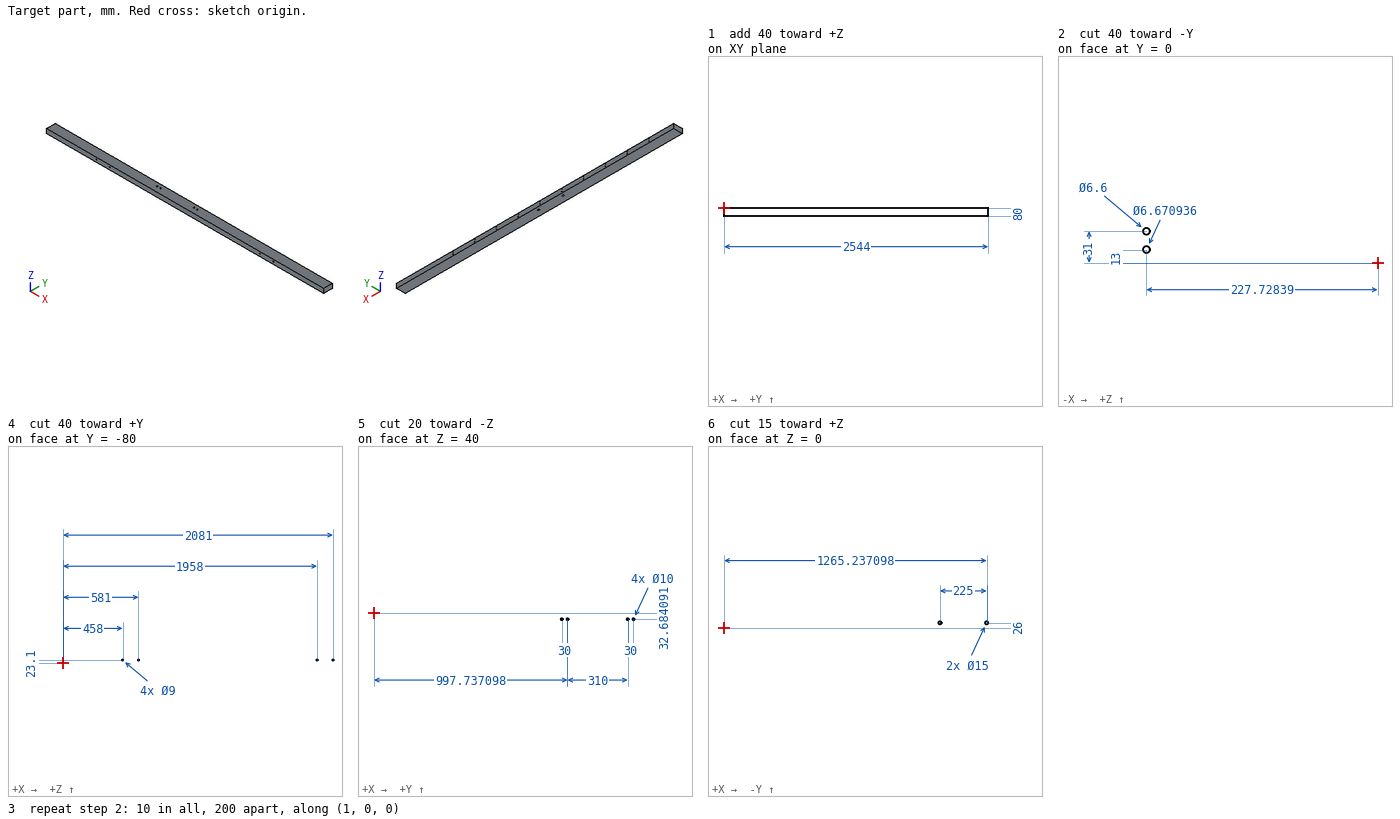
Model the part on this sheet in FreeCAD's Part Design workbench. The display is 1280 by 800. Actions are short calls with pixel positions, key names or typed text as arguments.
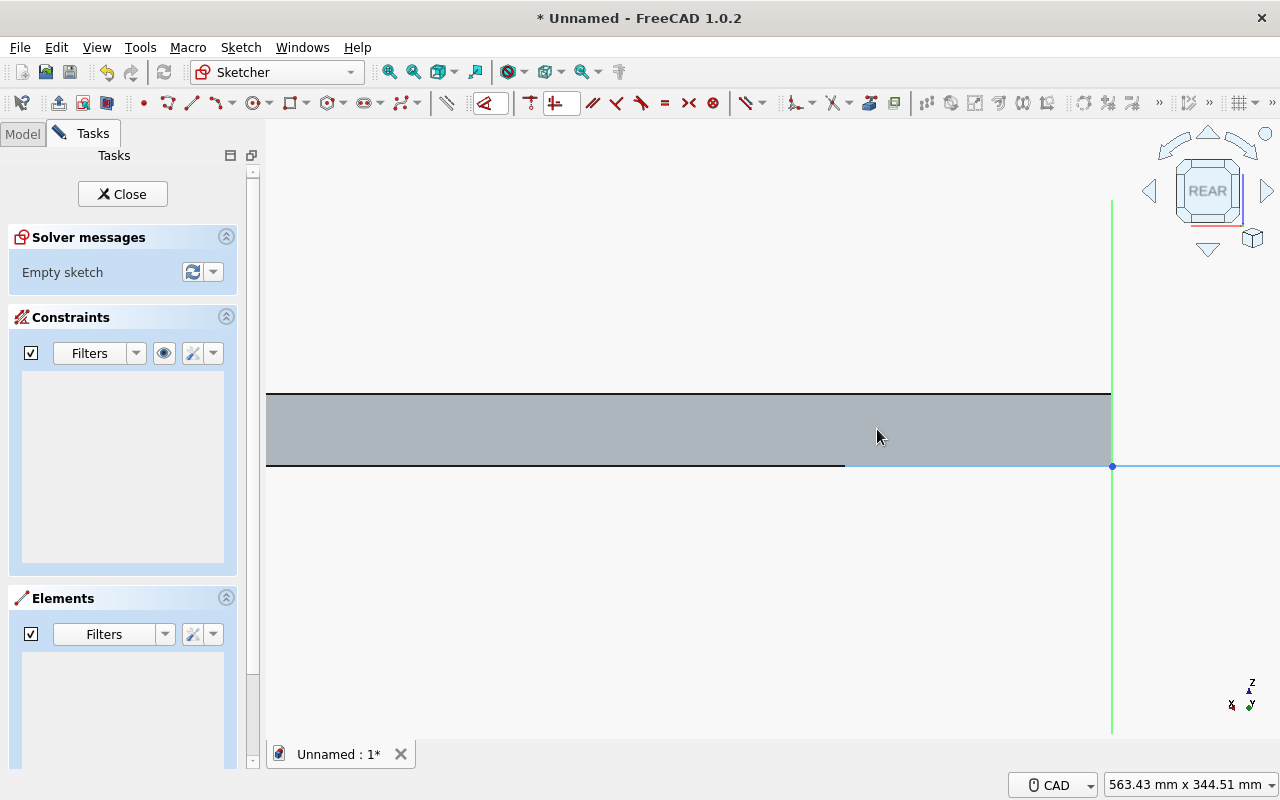
scroll(702, 427, up, 11)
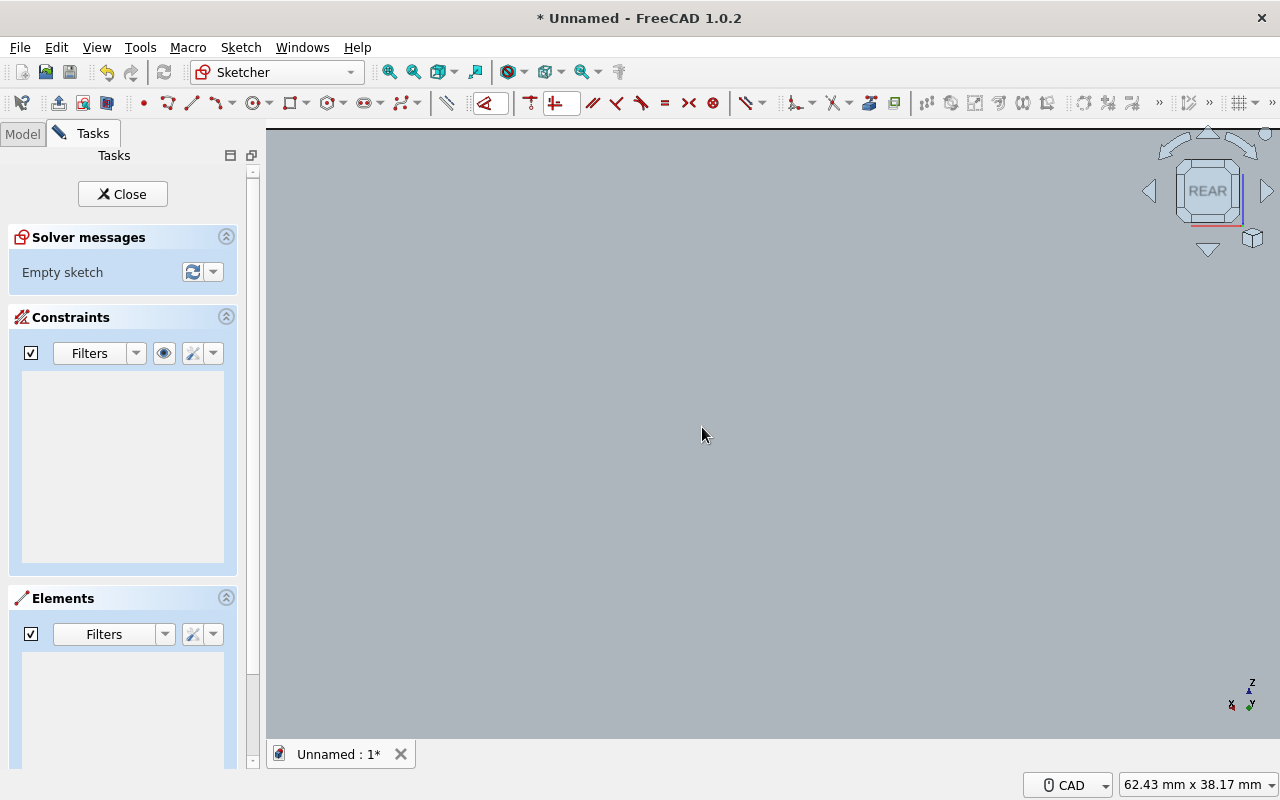
click(254, 104)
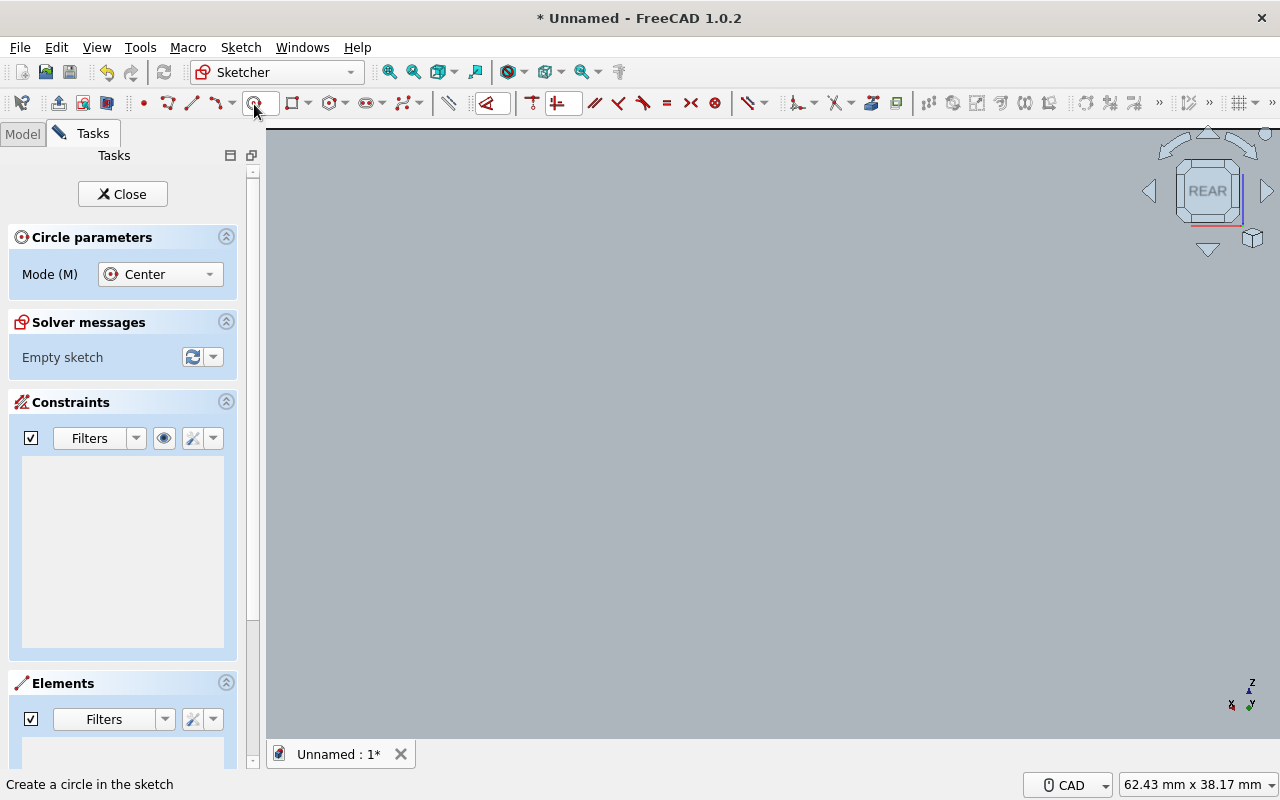
click(702, 568)
move(741, 530)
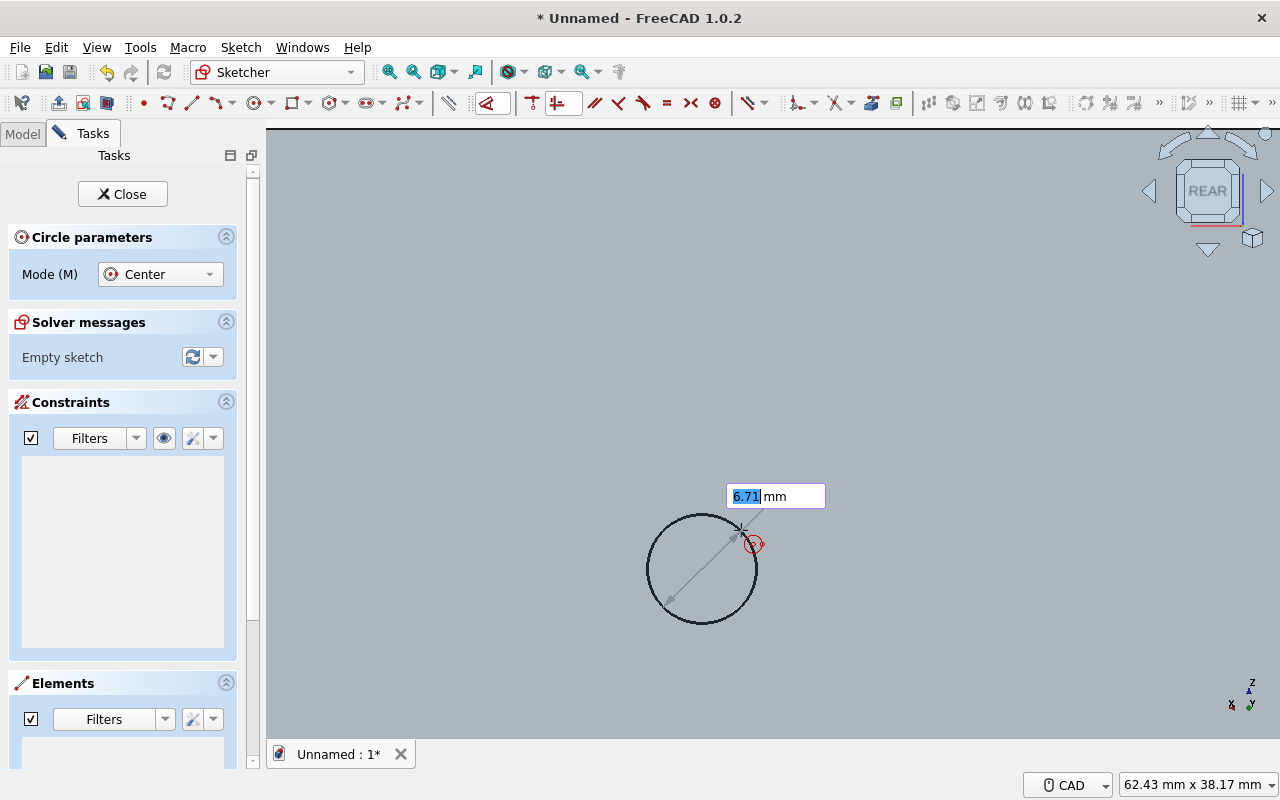
text(6.670936)
key(Return)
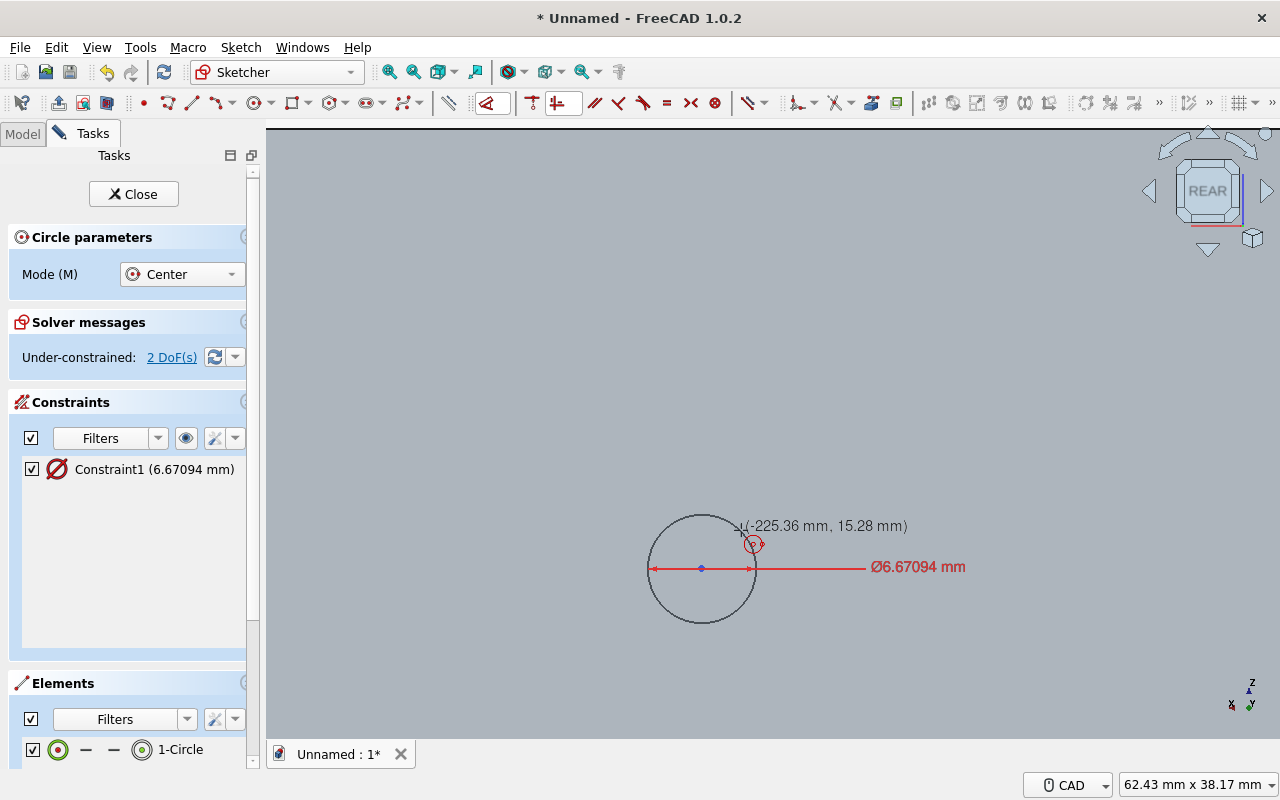
click(702, 276)
move(740, 238)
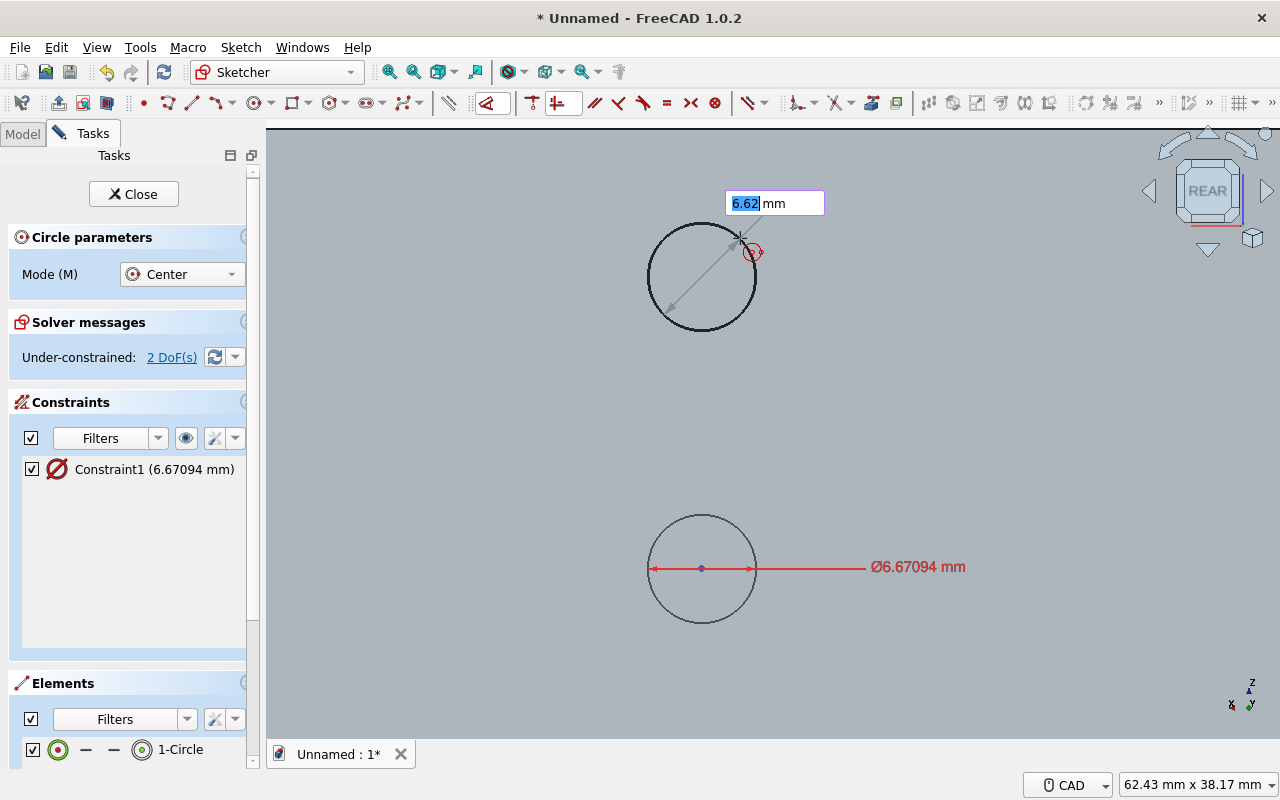
text(6.6)
key(Return)
key(Escape)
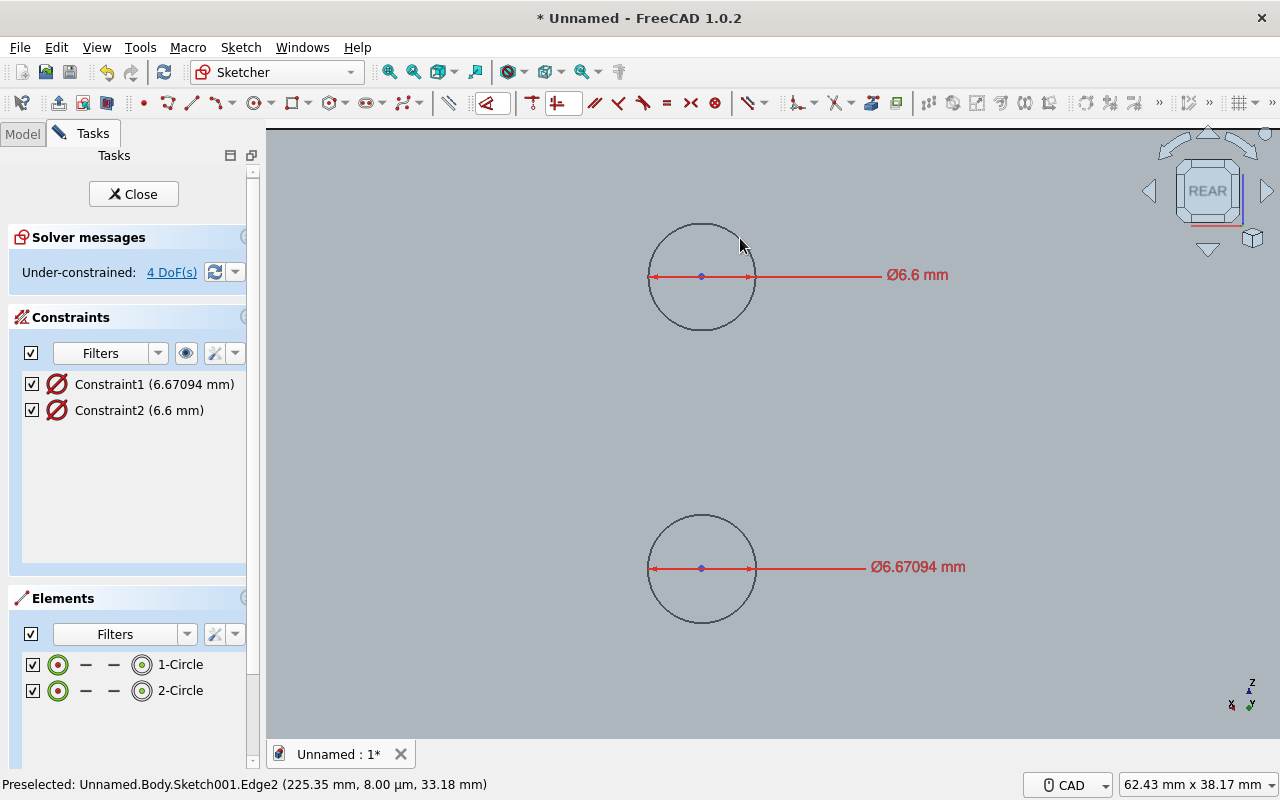
click(702, 569)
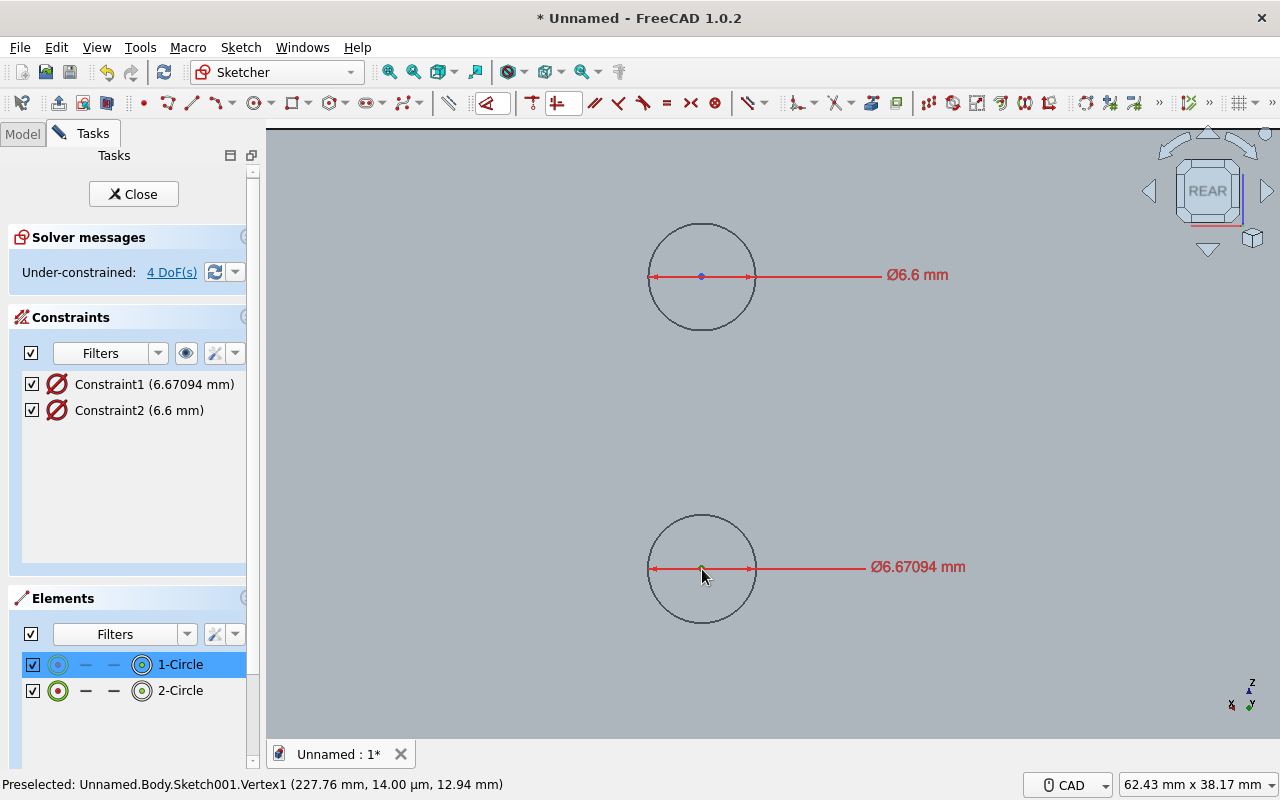
click(702, 277)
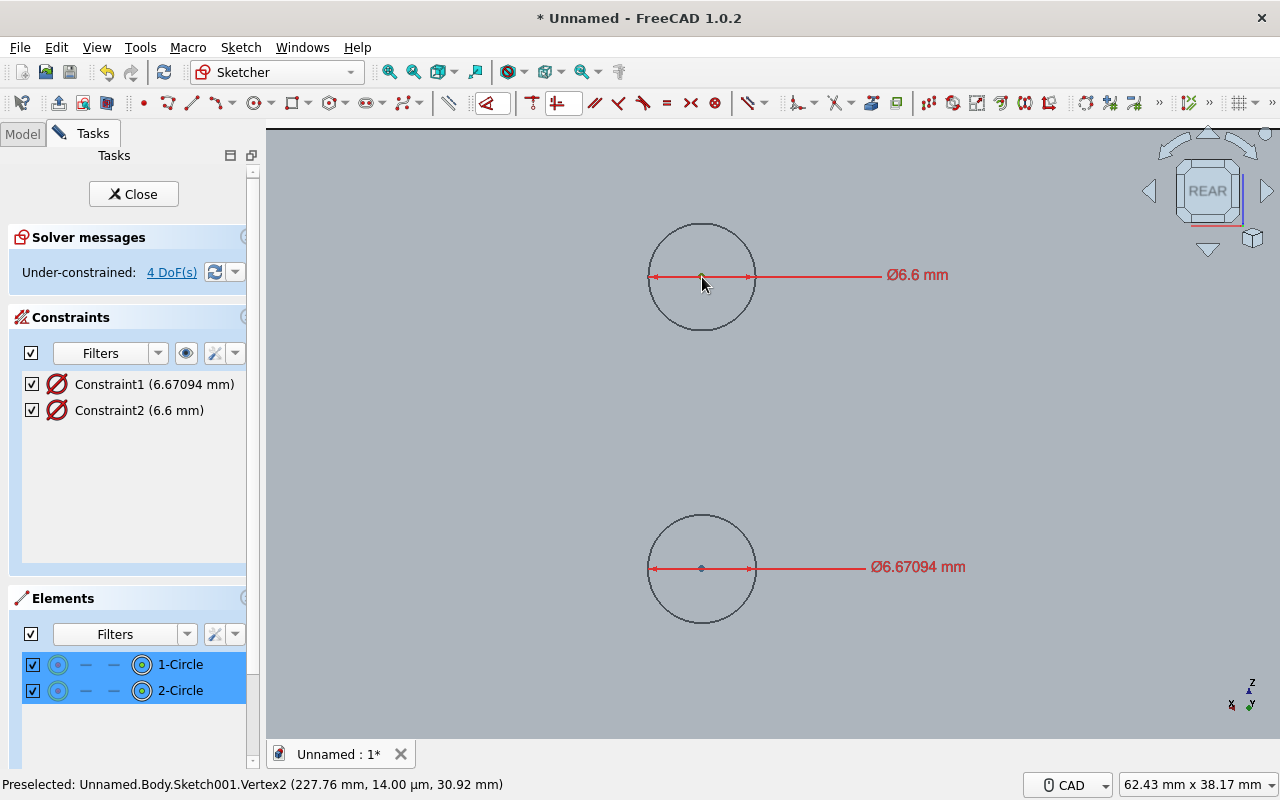
key(v)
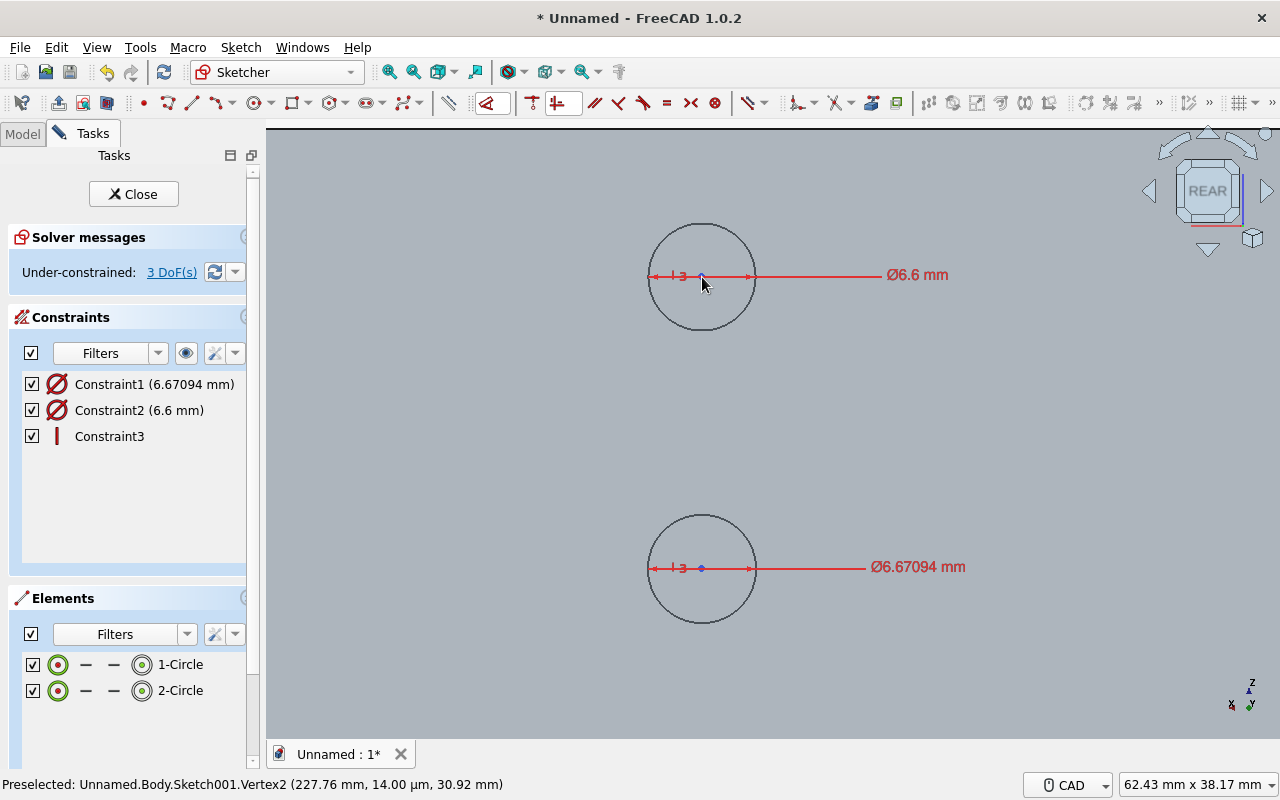
key(d)